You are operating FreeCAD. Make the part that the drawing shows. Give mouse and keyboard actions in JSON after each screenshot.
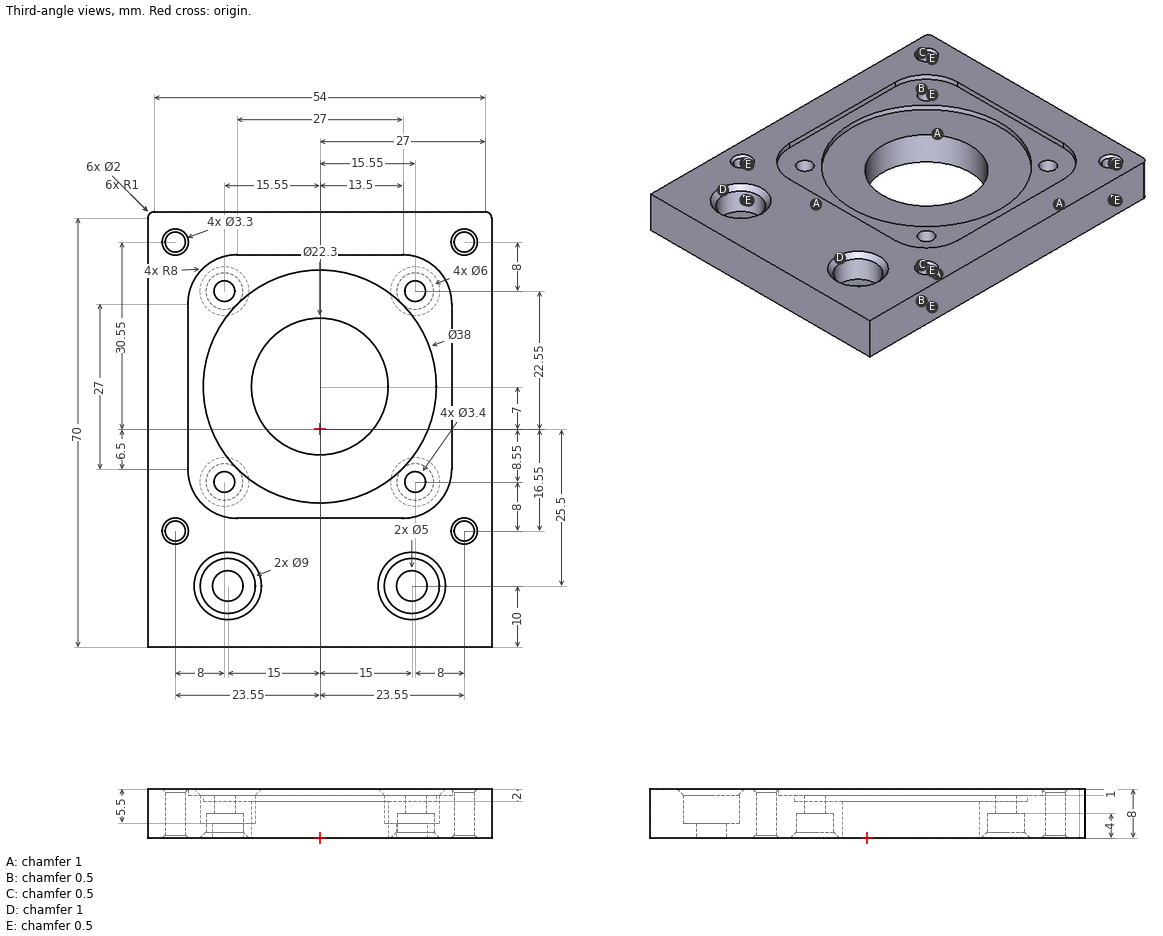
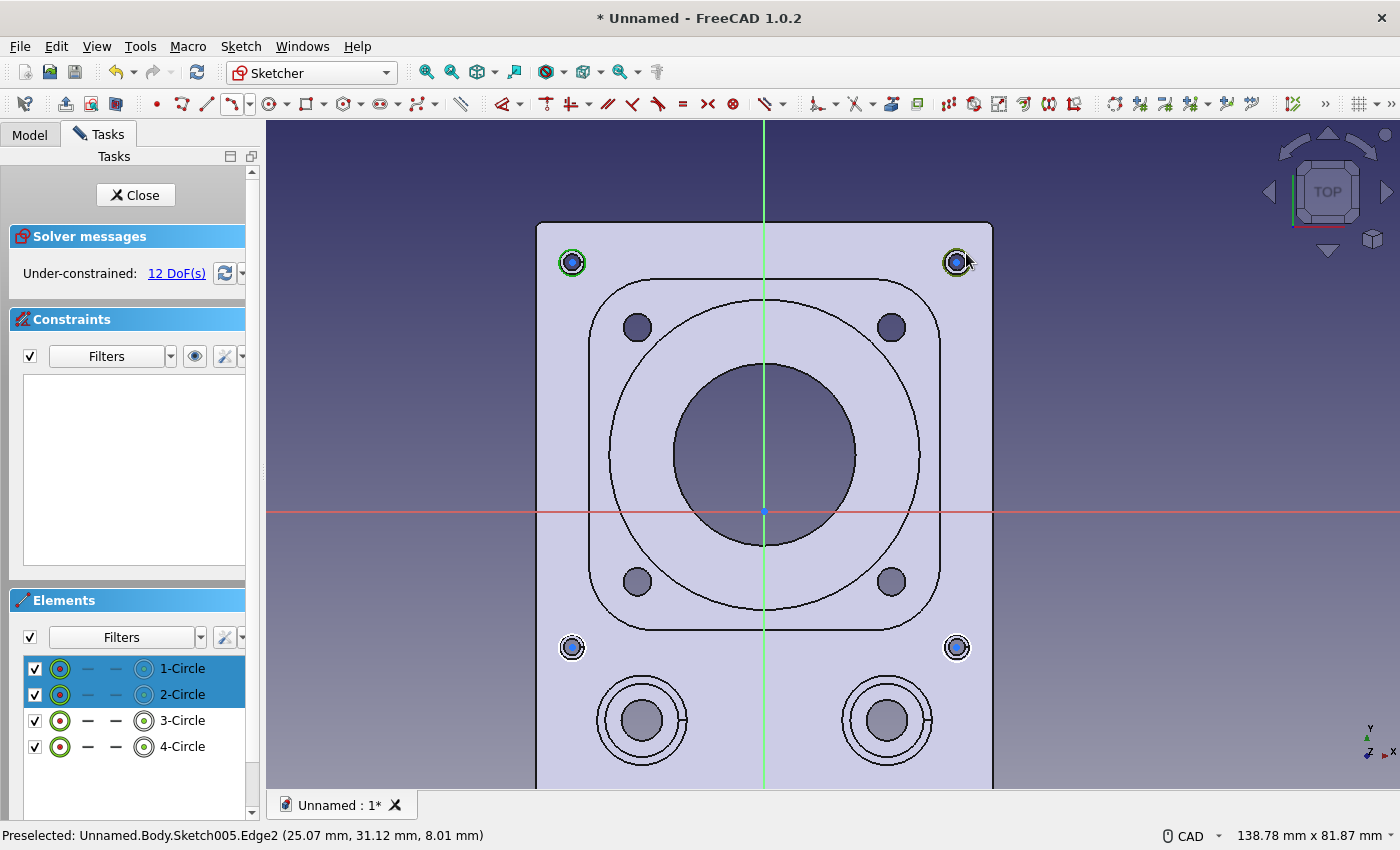
{"action": "left_click", "coordinate": [967, 638]}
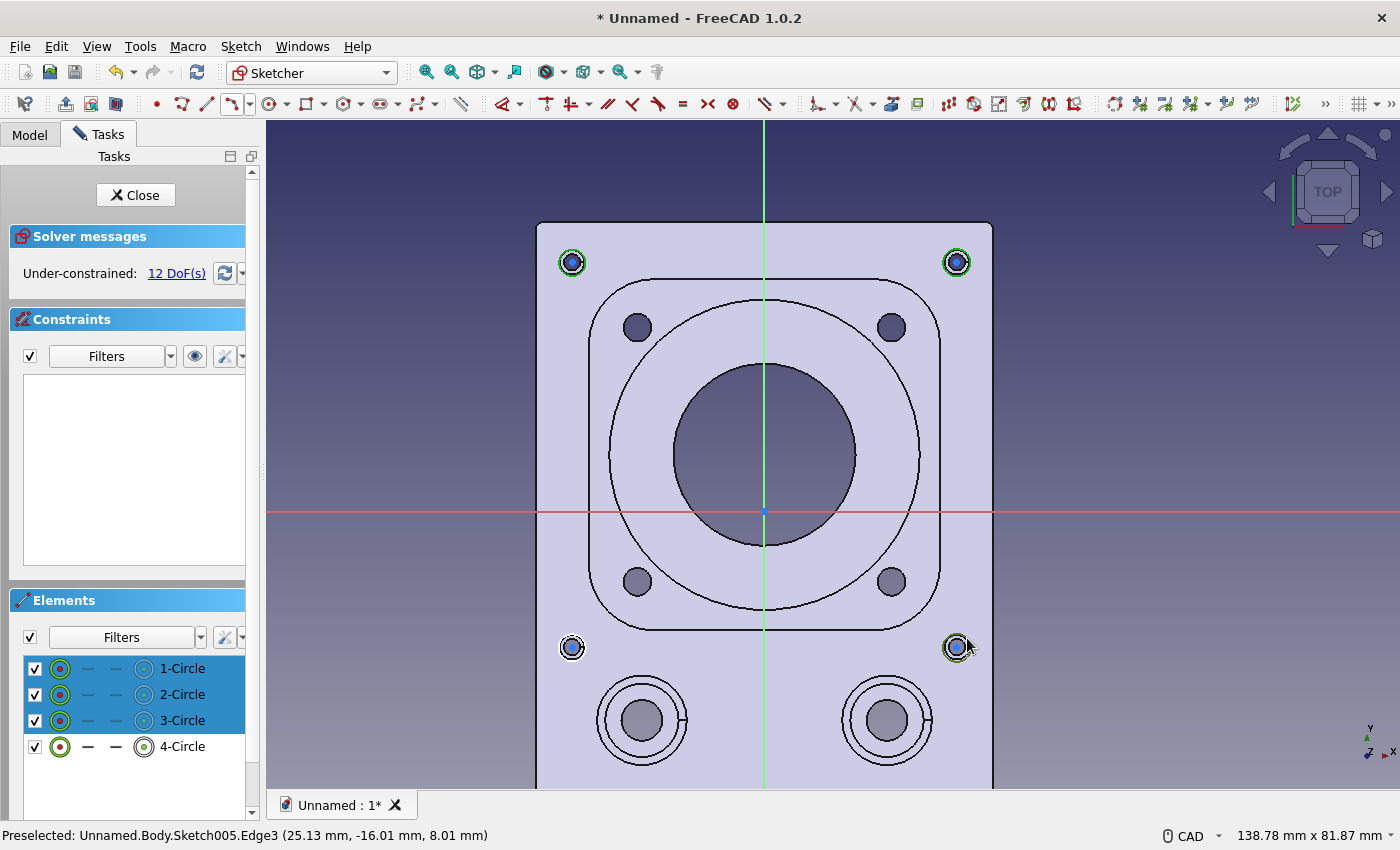
{"action": "left_click", "coordinate": [582, 638]}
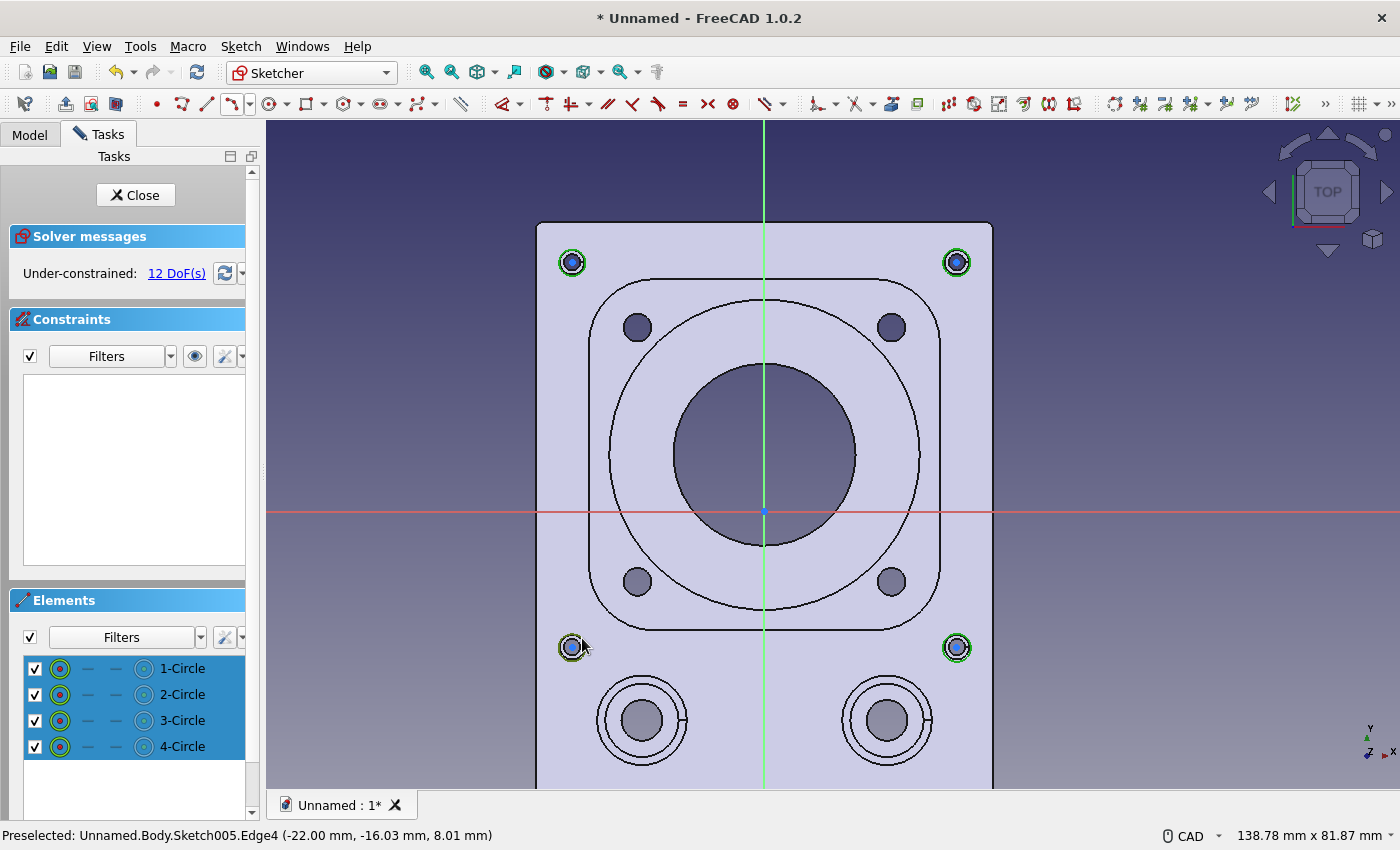
{"action": "left_click", "coordinate": [683, 104]}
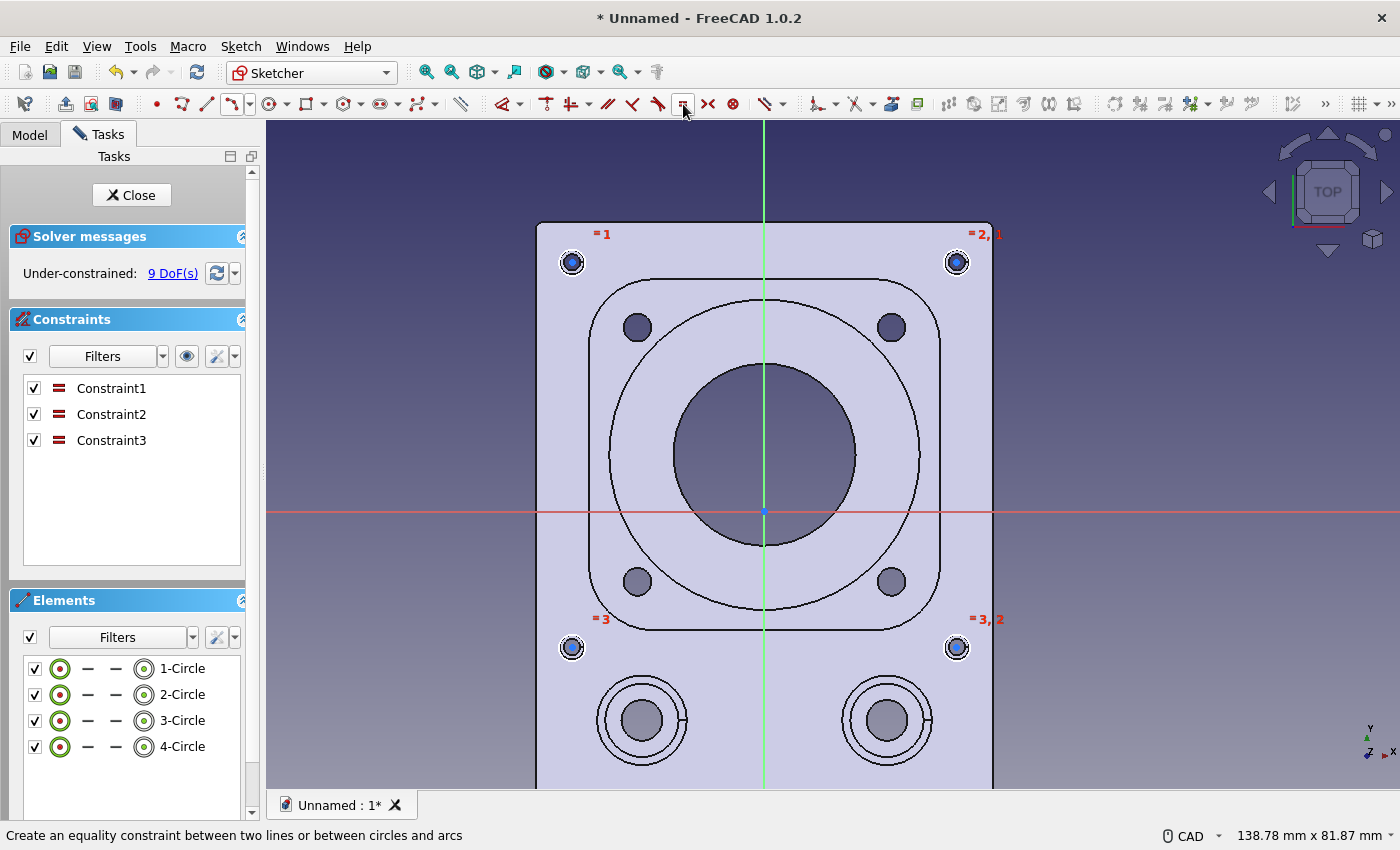
{"action": "key", "text": "d"}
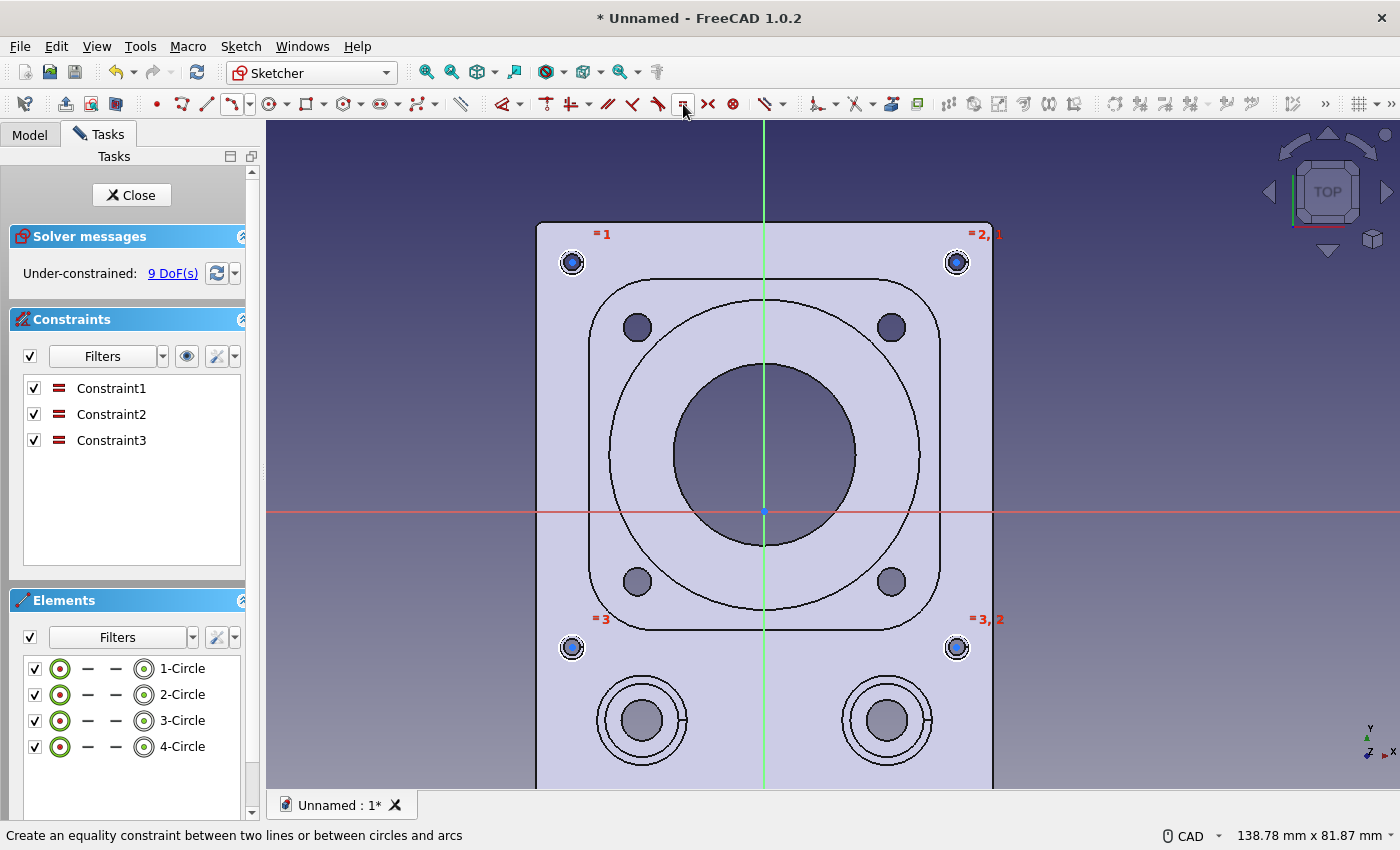
{"action": "scroll", "coordinate": [582, 253], "scroll_direction": "up", "scroll_amount": 2}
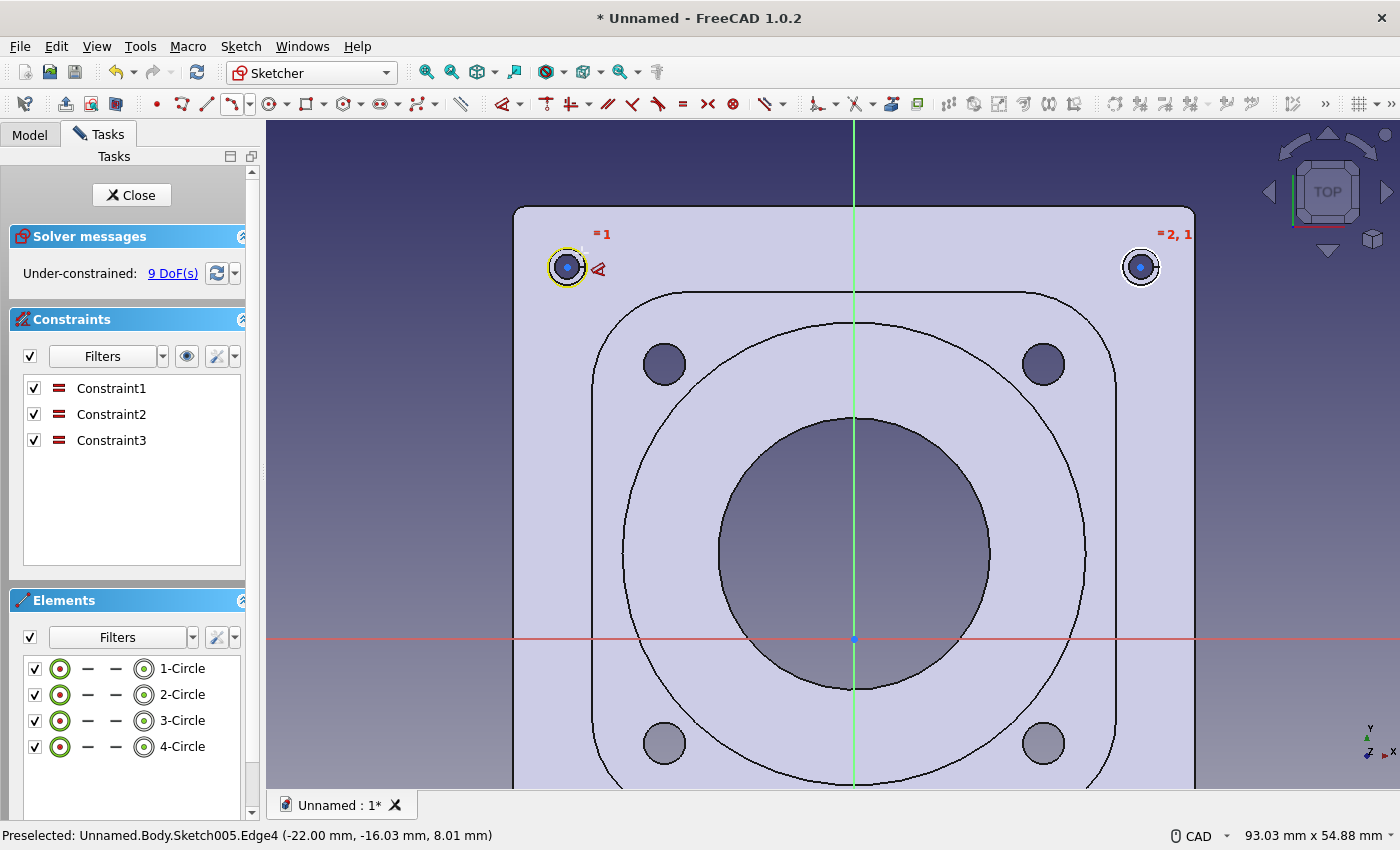
{"action": "left_click", "coordinate": [581, 254]}
{"action": "left_click", "coordinate": [604, 231]}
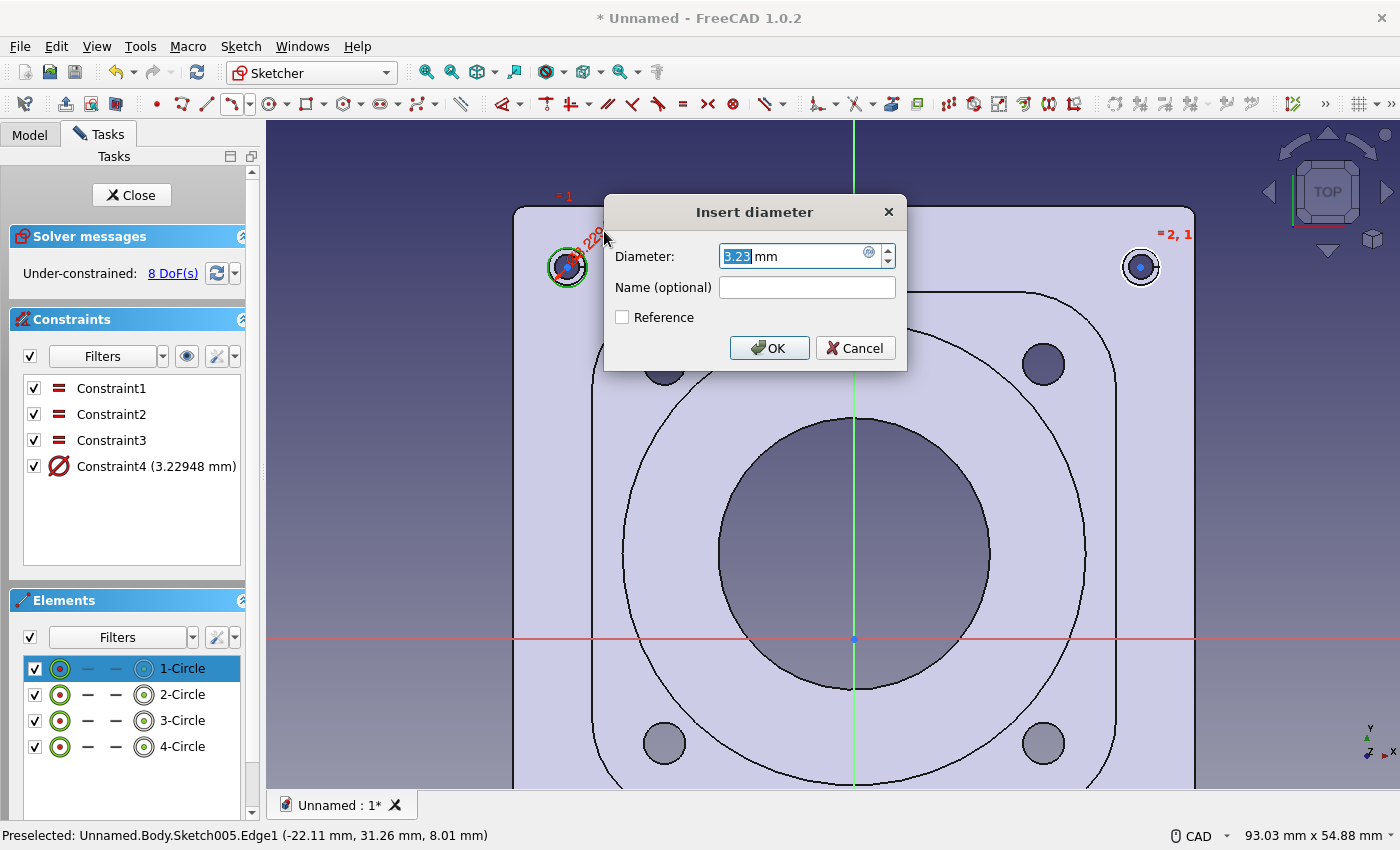
{"action": "type", "text": "3.3"}
{"action": "key", "text": "Return"}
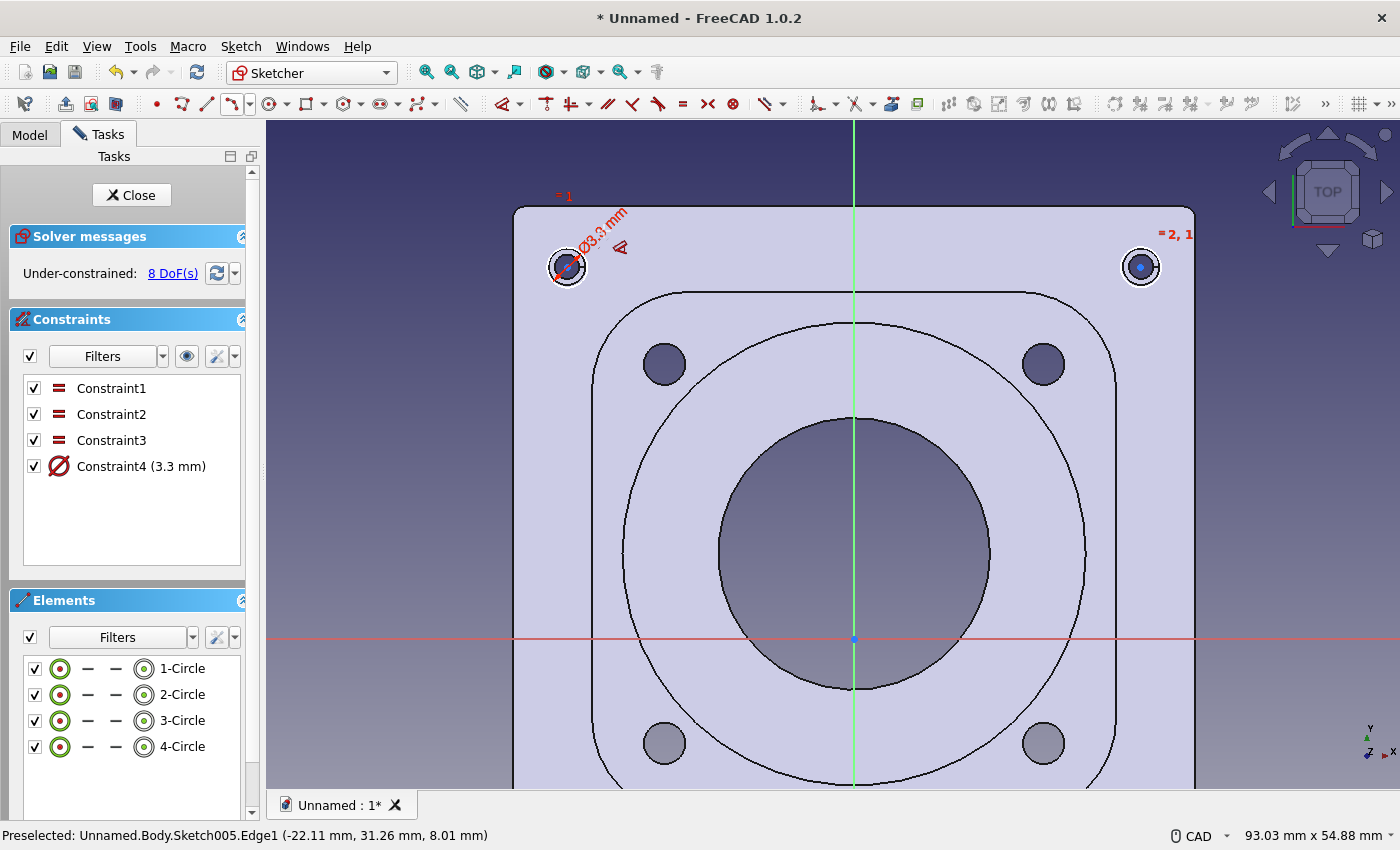
{"action": "left_click", "coordinate": [567, 268]}
{"action": "left_click", "coordinate": [711, 234]}